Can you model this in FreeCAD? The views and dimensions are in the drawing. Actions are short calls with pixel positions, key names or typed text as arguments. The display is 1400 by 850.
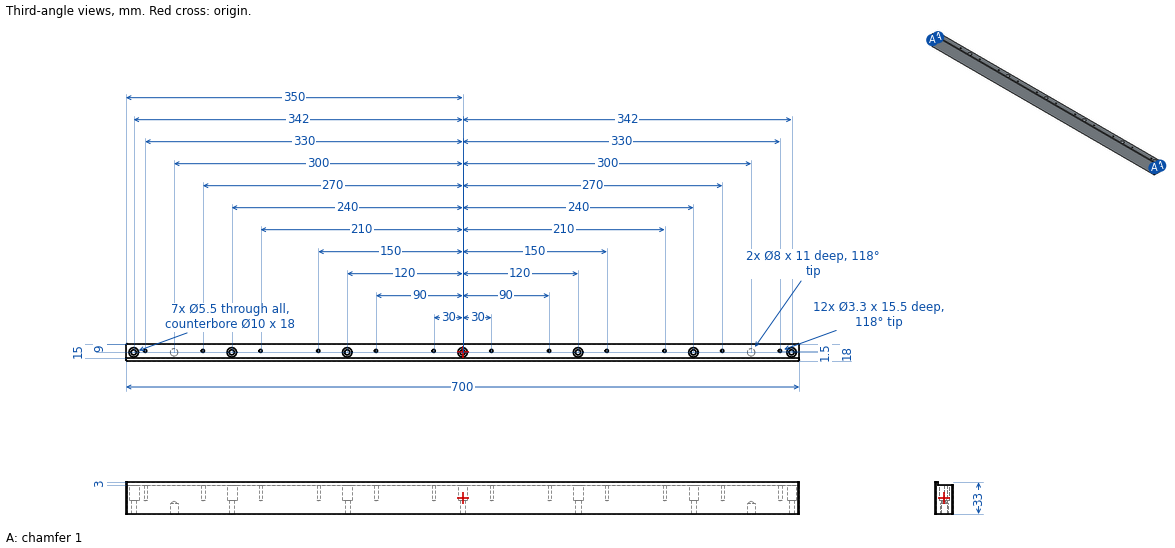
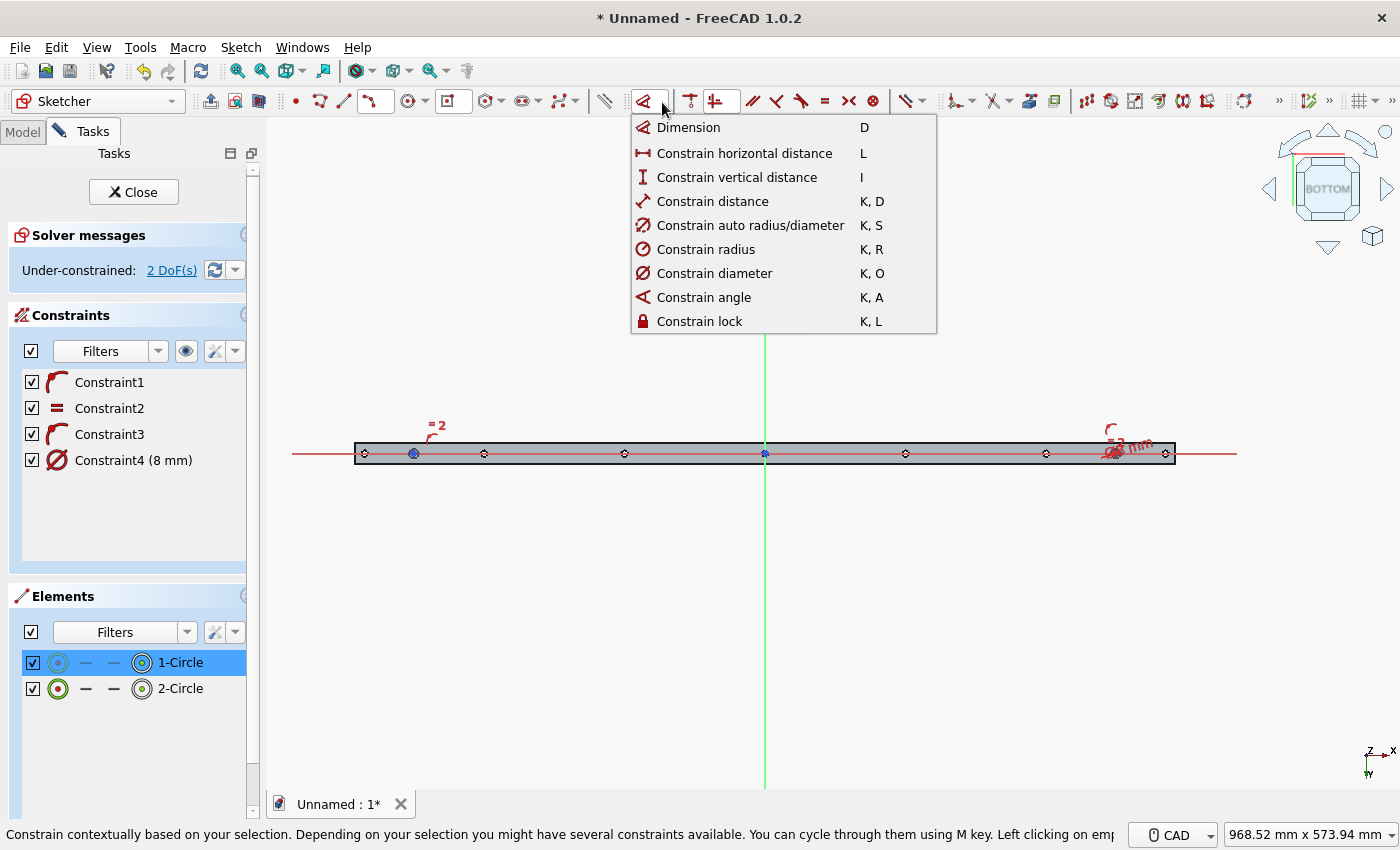
click(784, 153)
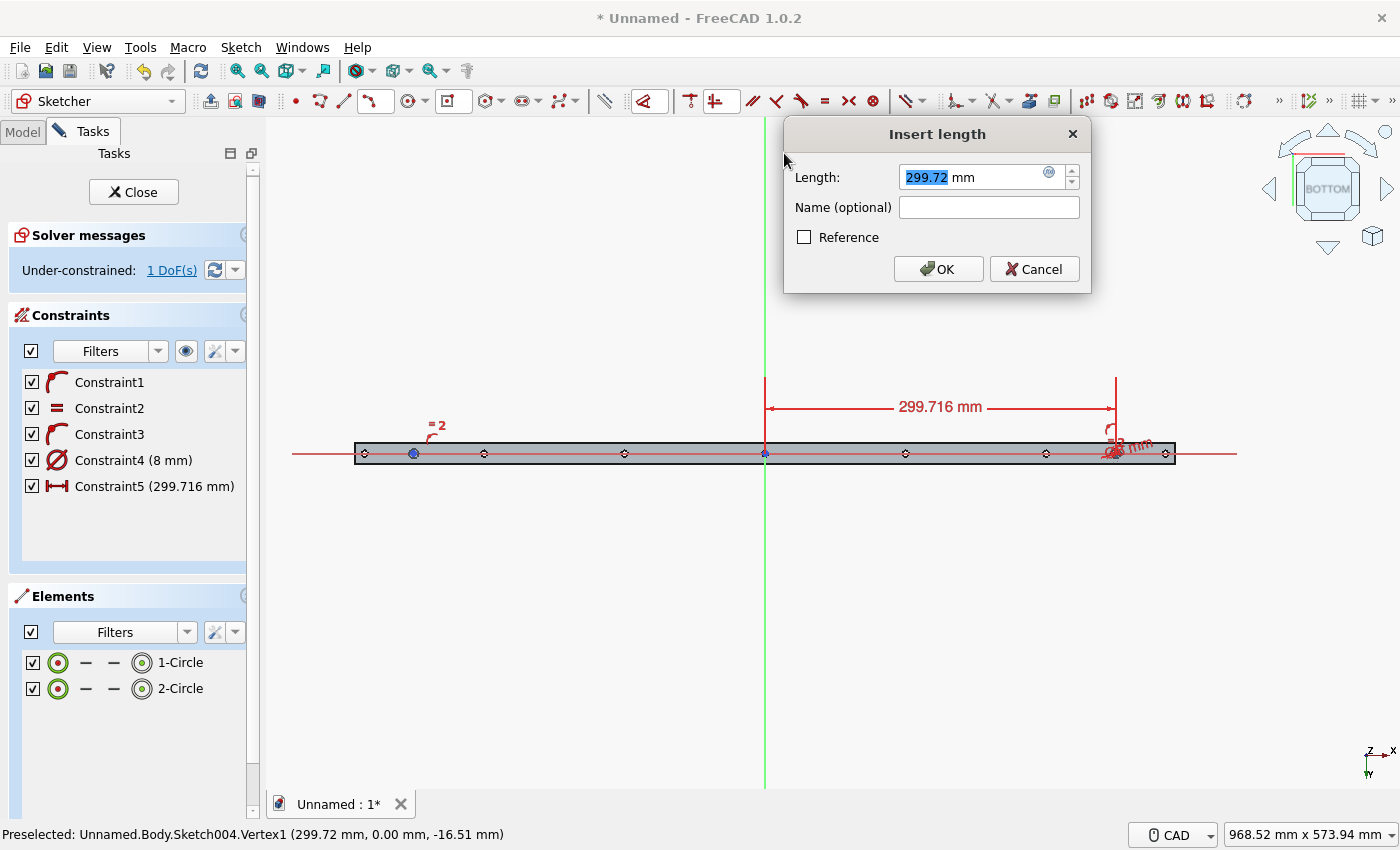
text(300)
key(Return)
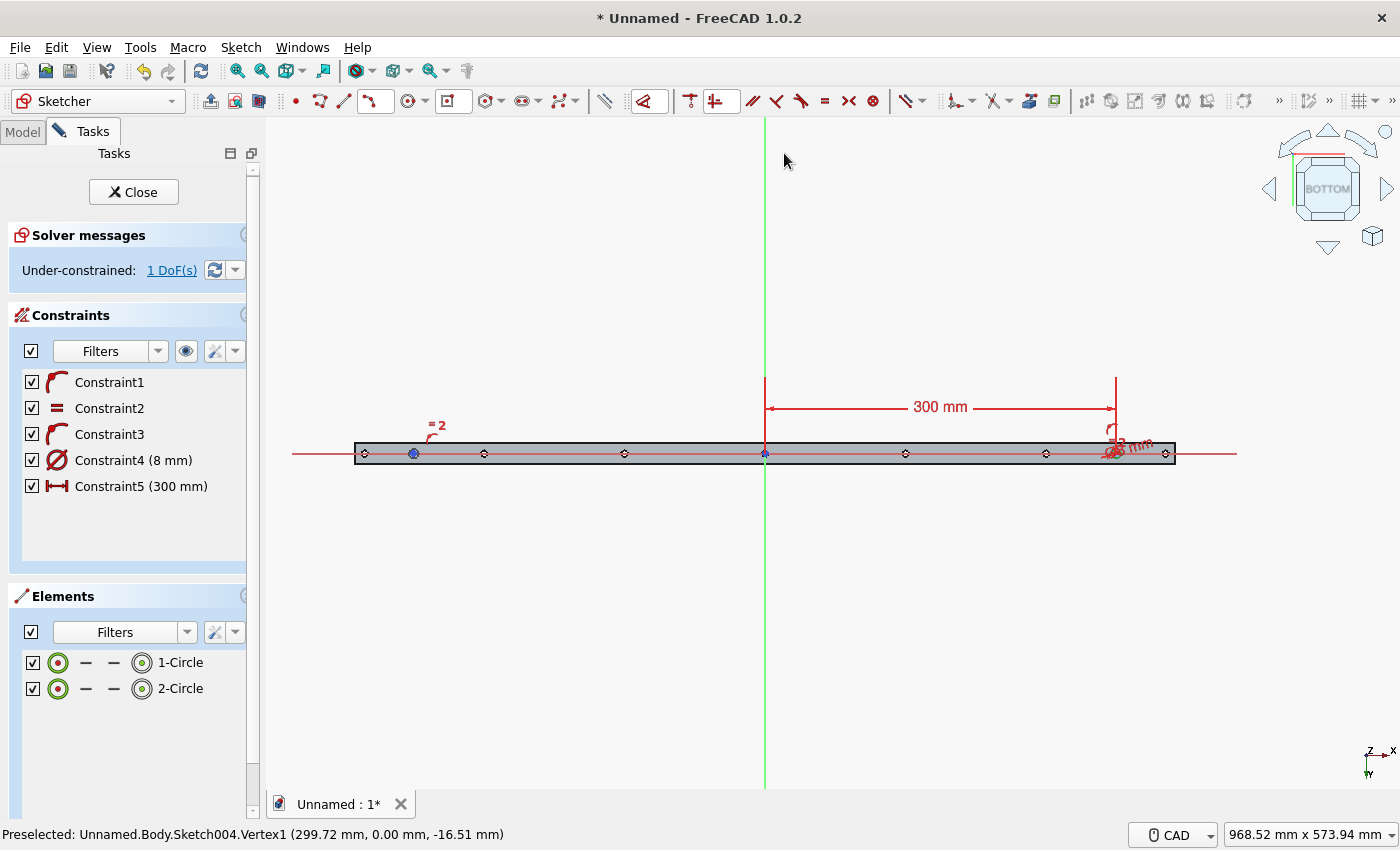
click(414, 454)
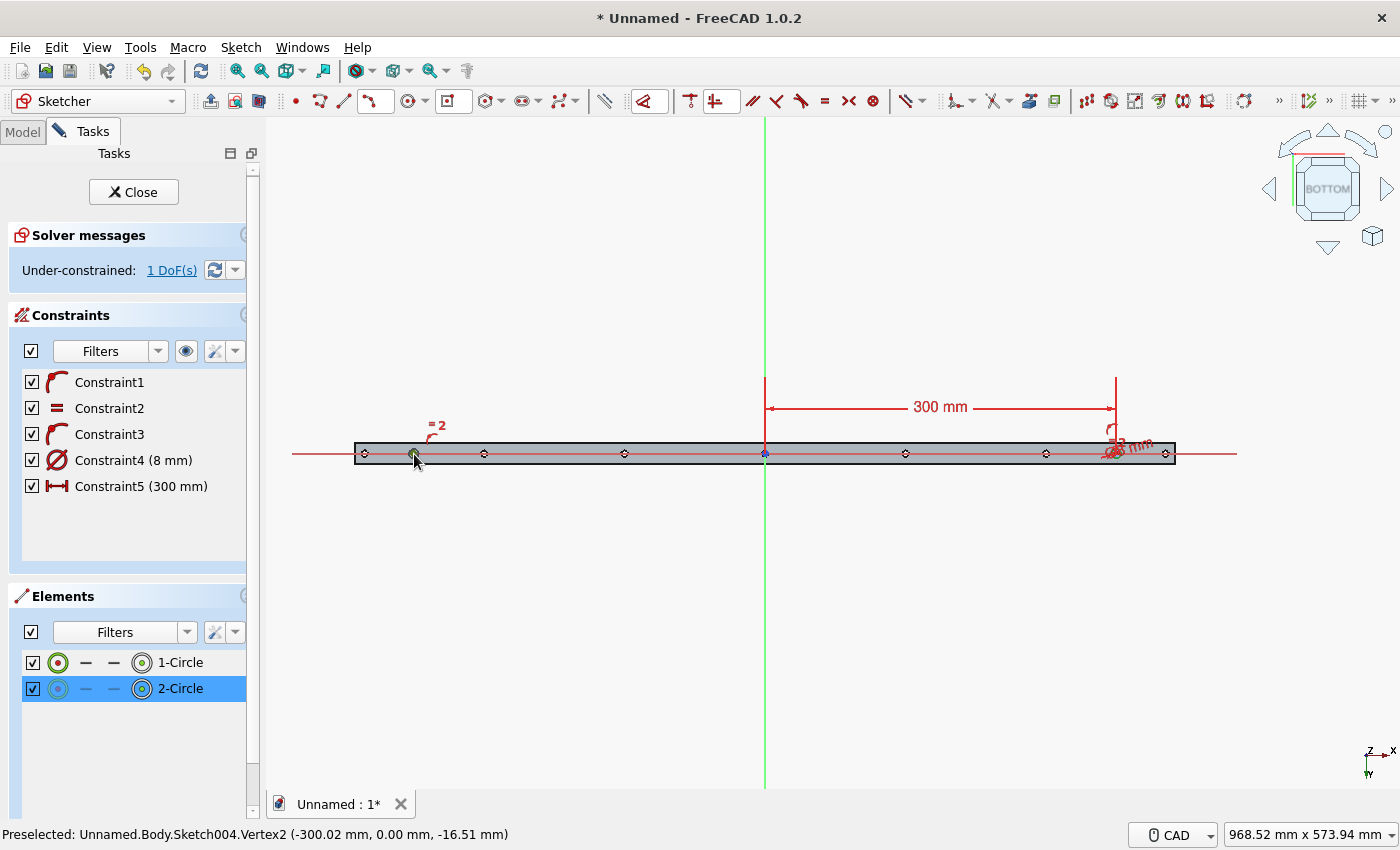
key(l)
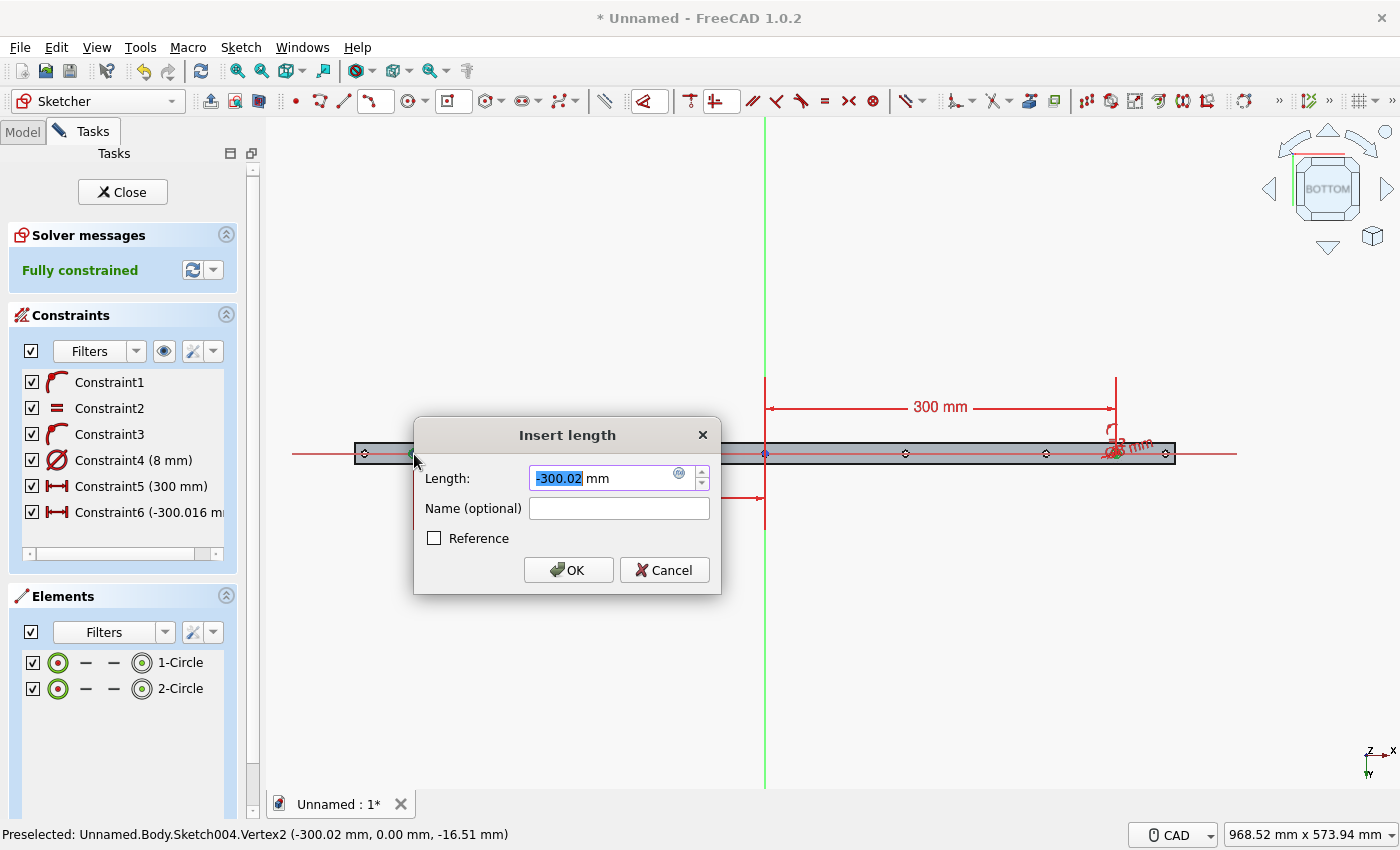
text(-300)
key(Return)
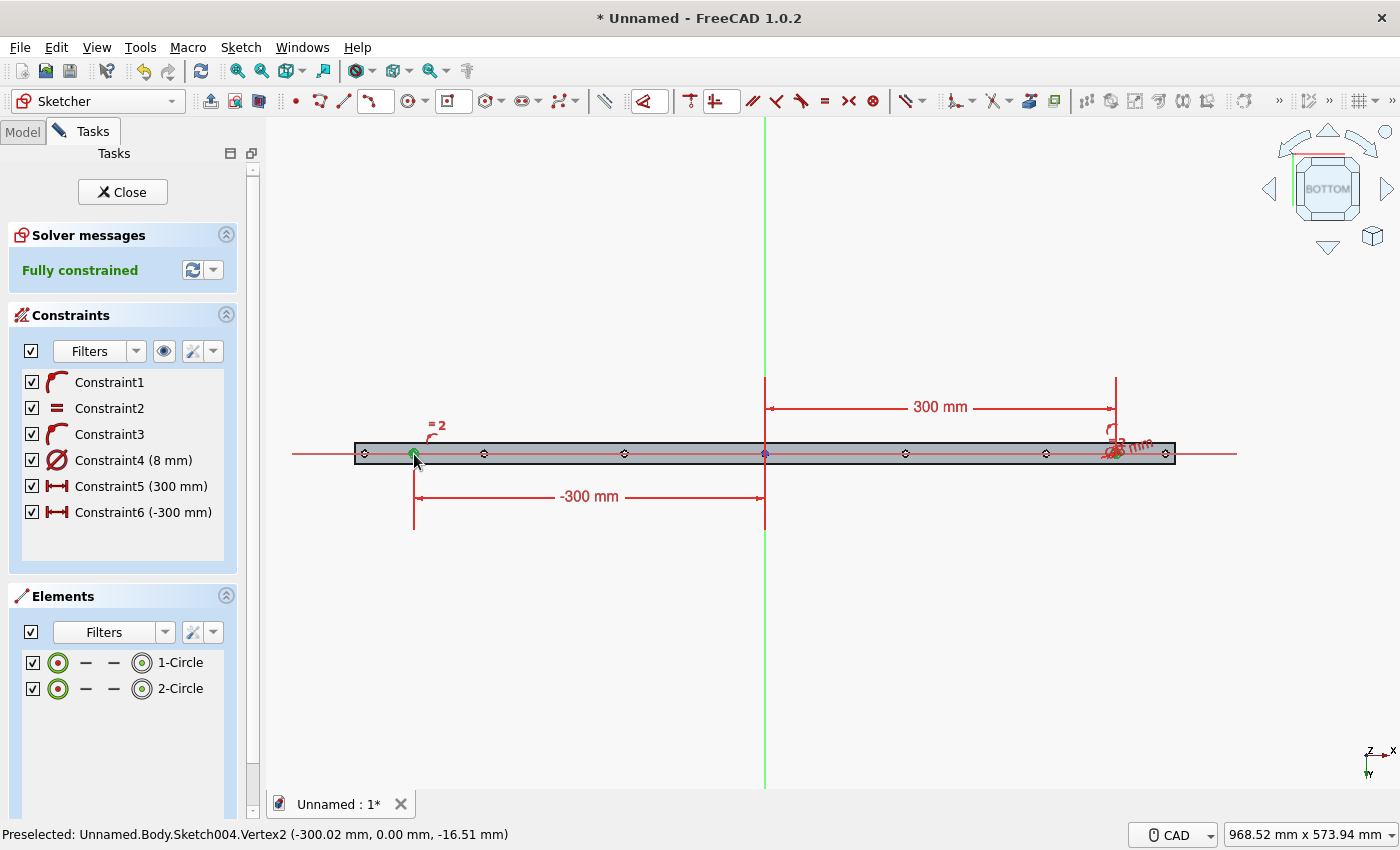
click(123, 192)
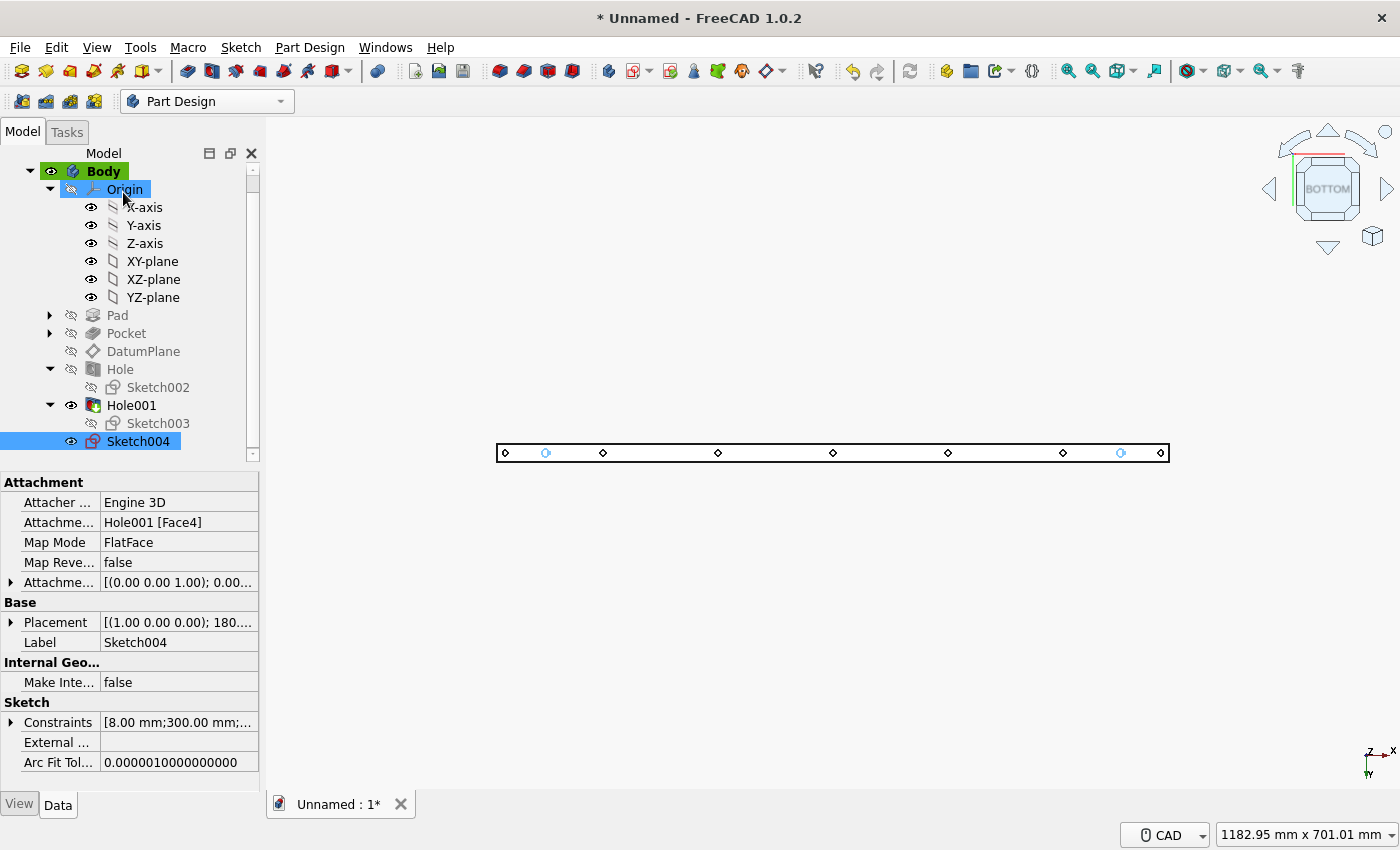
click(212, 72)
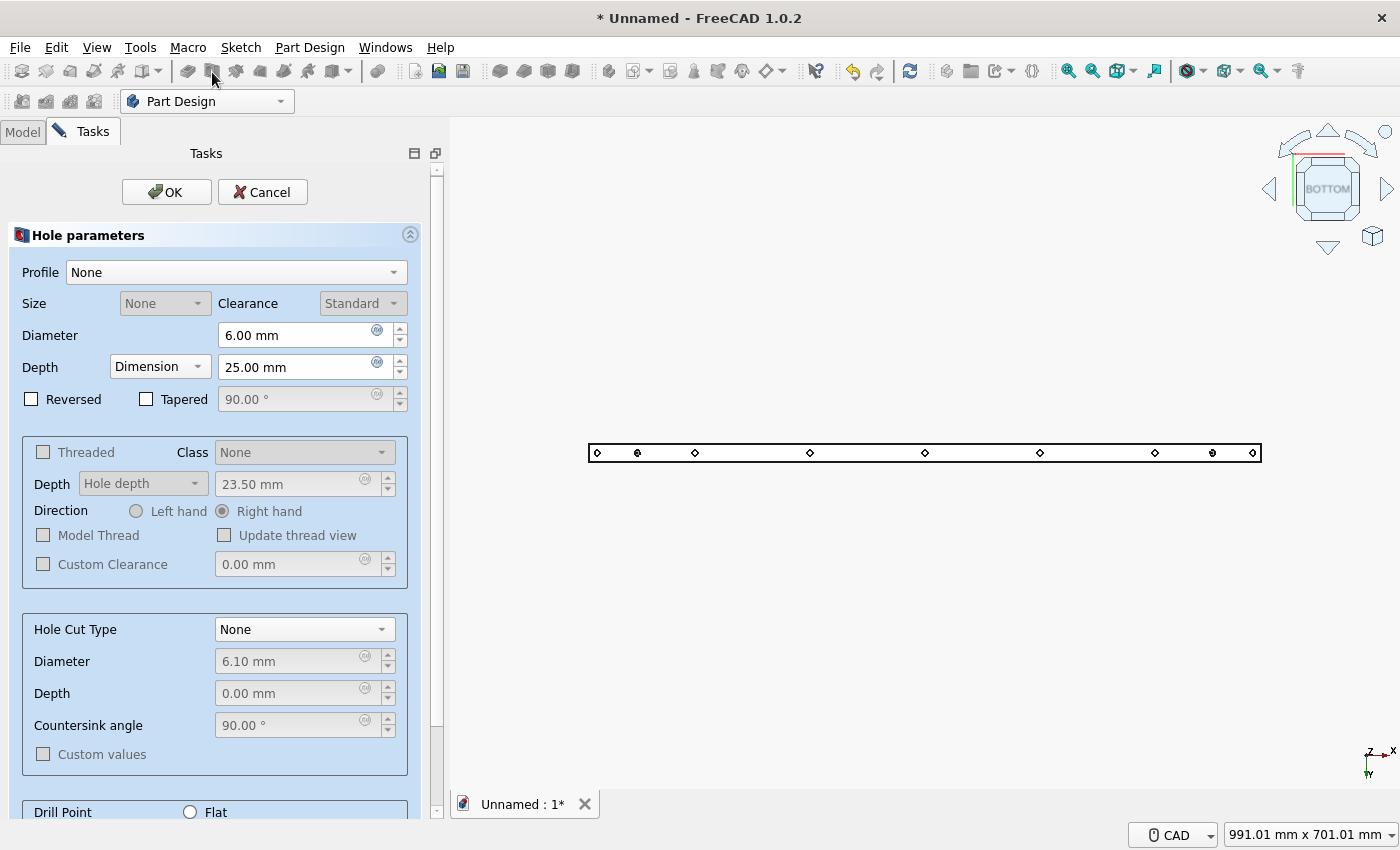
triple_click(305, 335)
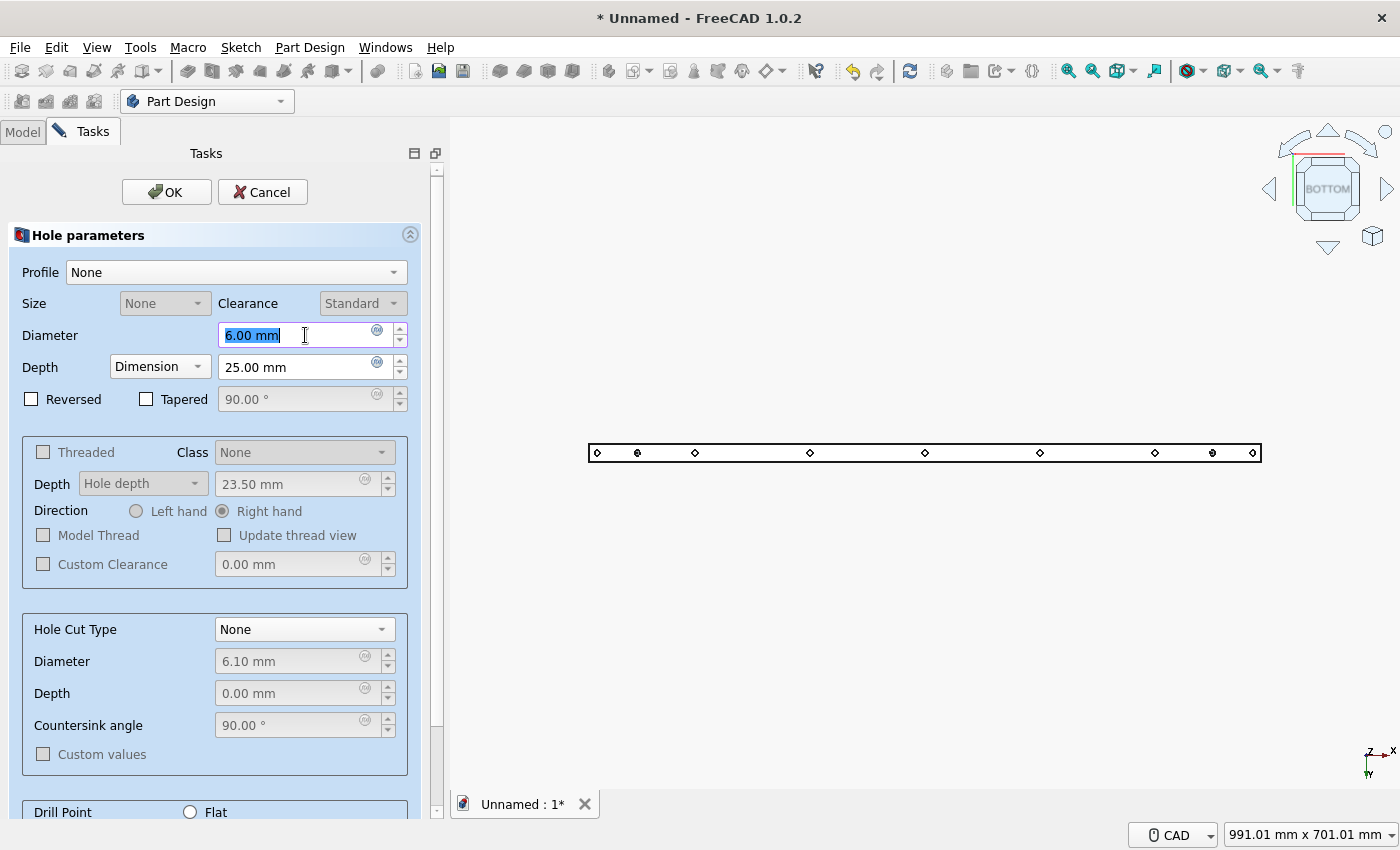
text(8)
key(Tab)